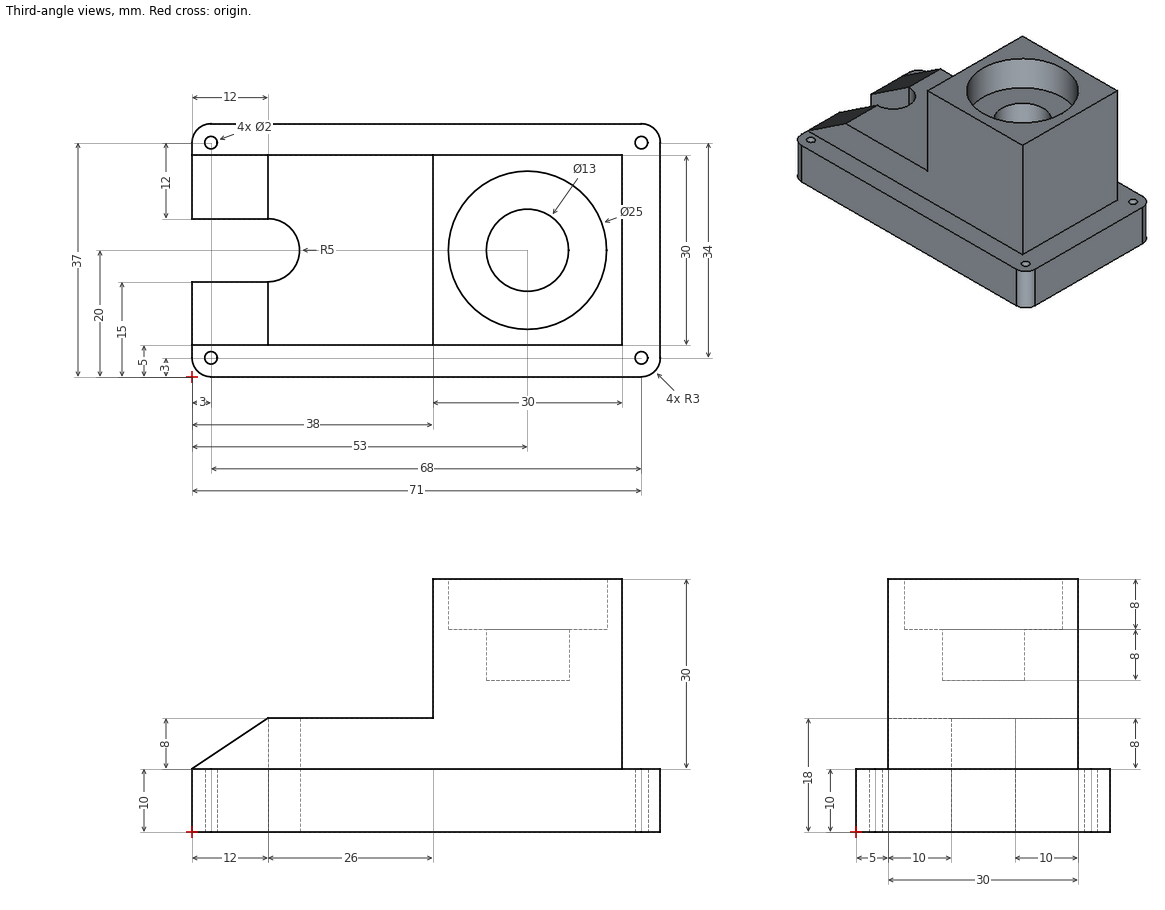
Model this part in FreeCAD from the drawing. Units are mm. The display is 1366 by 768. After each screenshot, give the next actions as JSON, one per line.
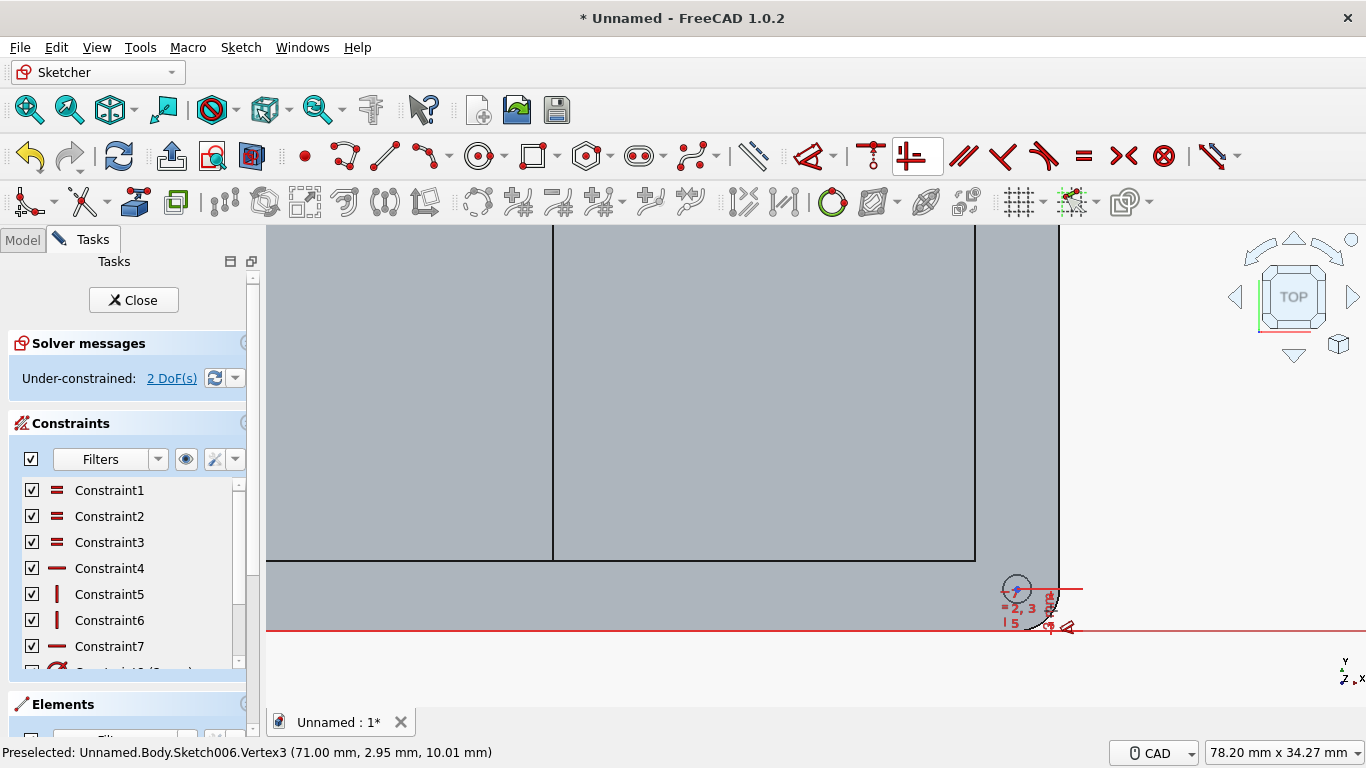
{"action": "scroll", "coordinate": [1018, 590], "scroll_direction": "down", "scroll_amount": 3}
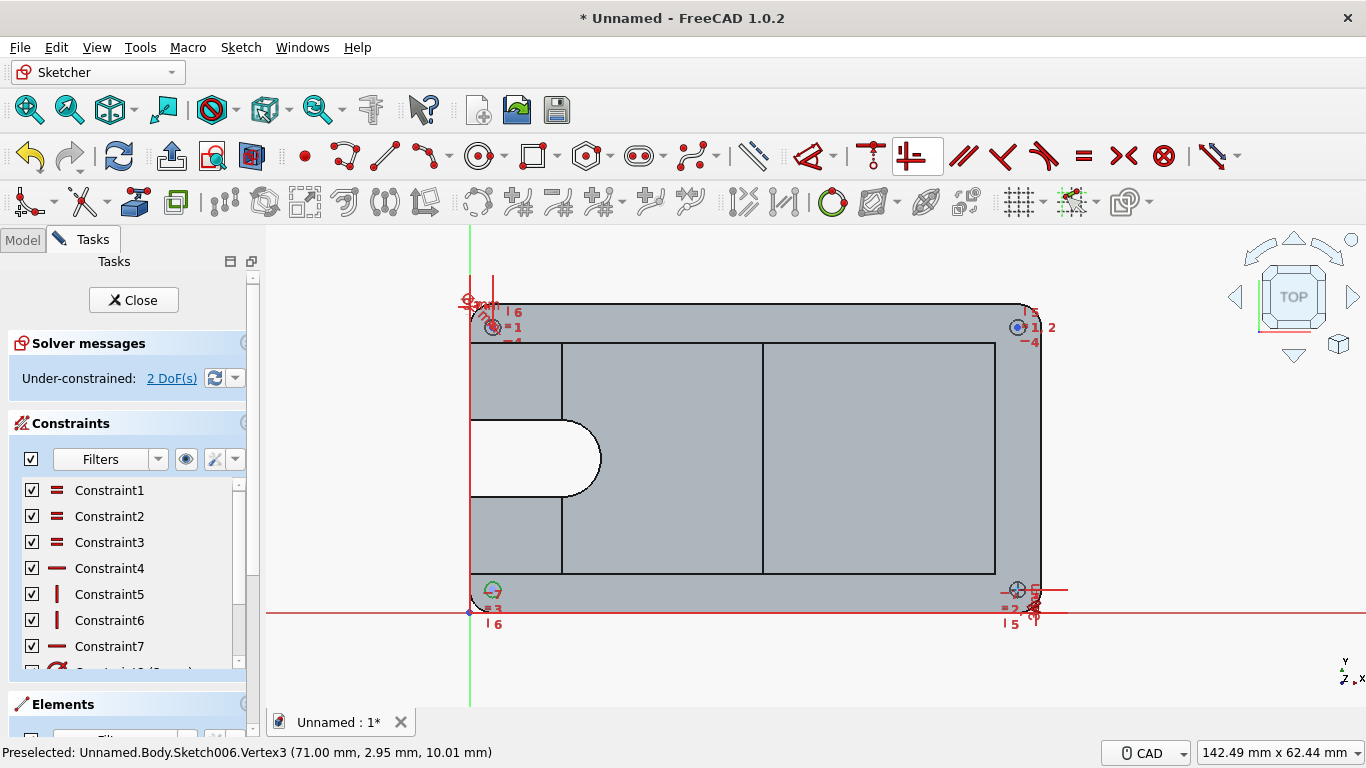
{"action": "left_click", "coordinate": [493, 328]}
{"action": "left_click", "coordinate": [436, 470]}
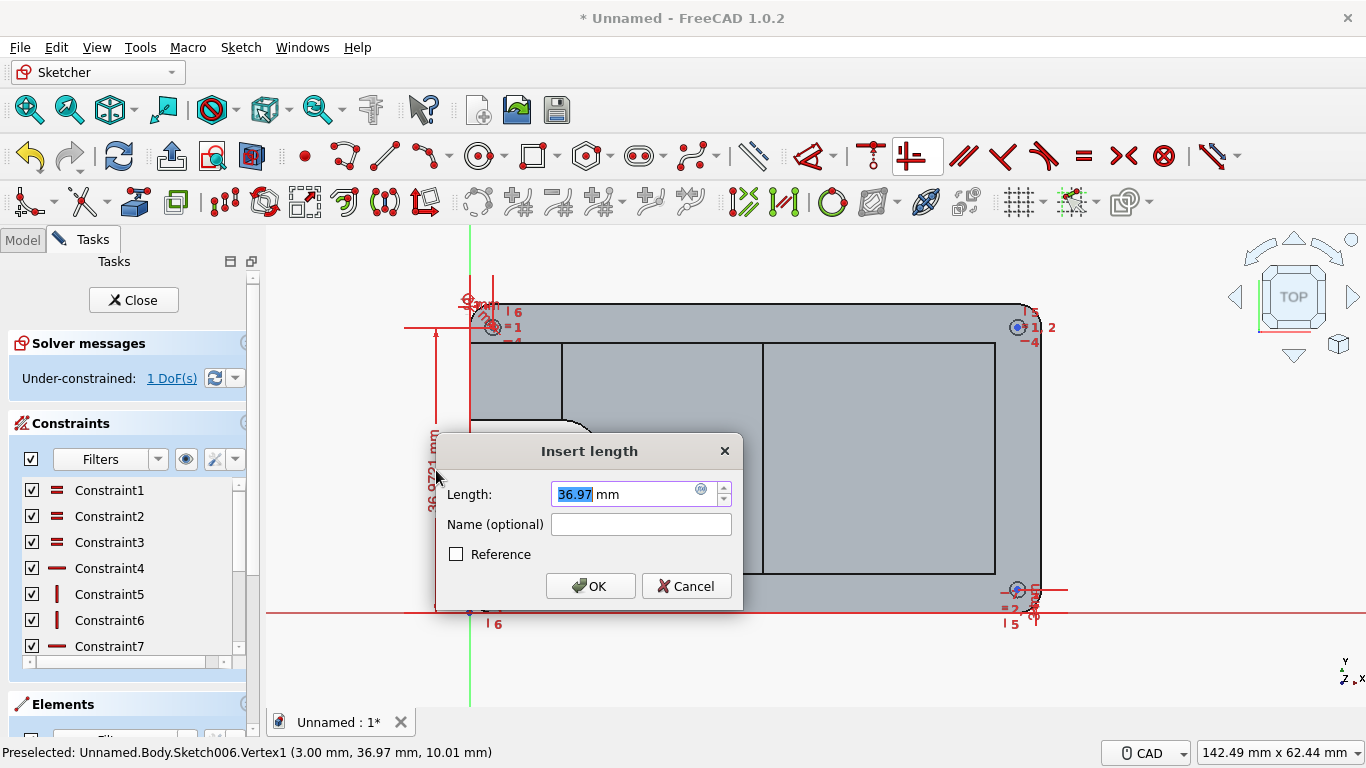
{"action": "type", "text": "37"}
{"action": "key", "text": "Return"}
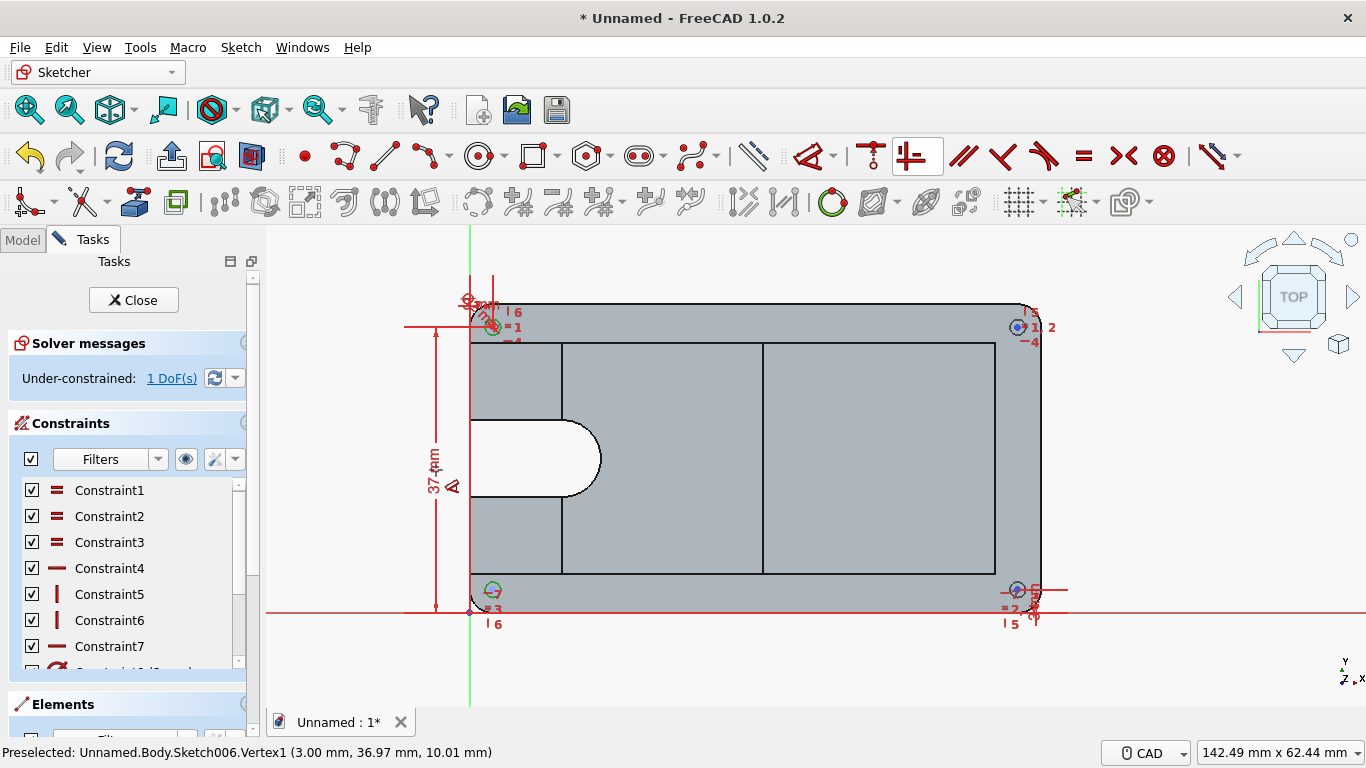
{"action": "left_click", "coordinate": [1018, 327]}
{"action": "left_click", "coordinate": [744, 647]}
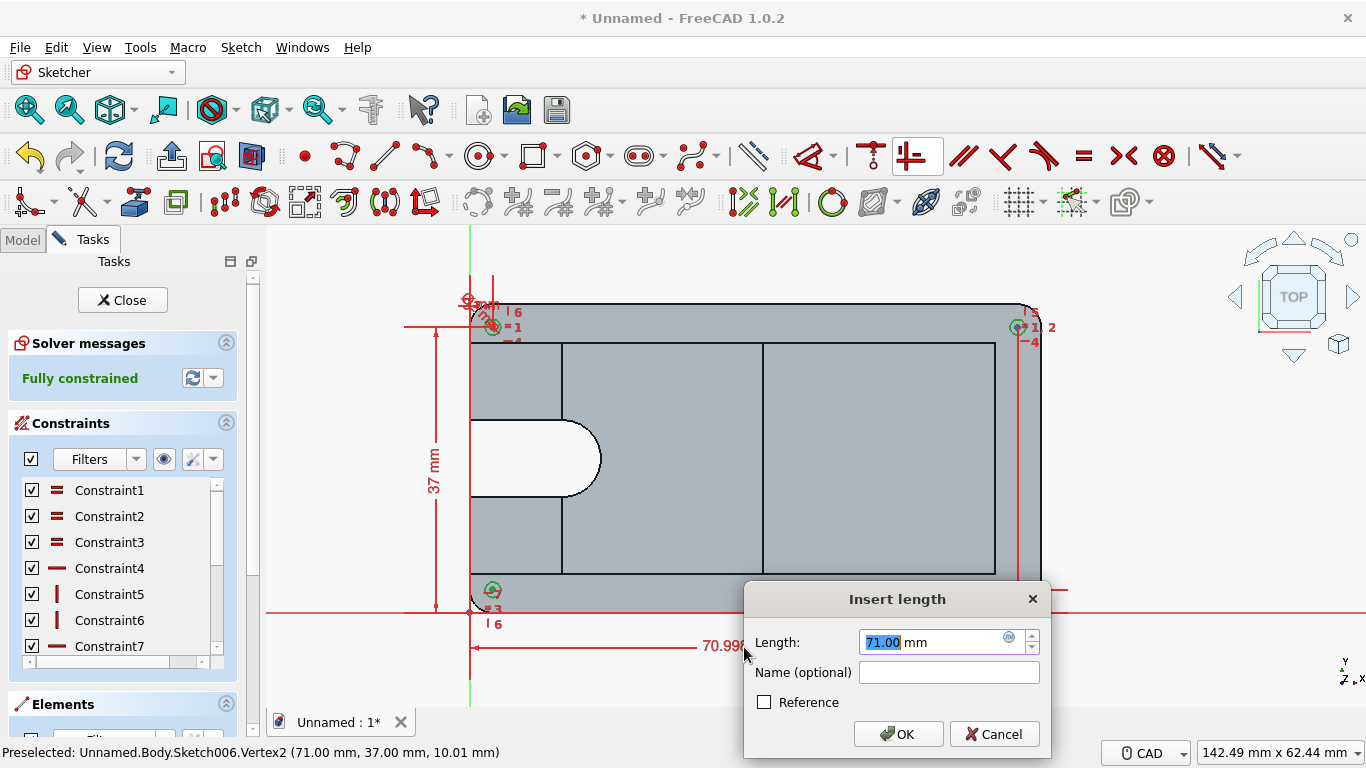
{"action": "type", "text": "71"}
{"action": "key", "text": "Return"}
{"action": "key", "text": "Escape"}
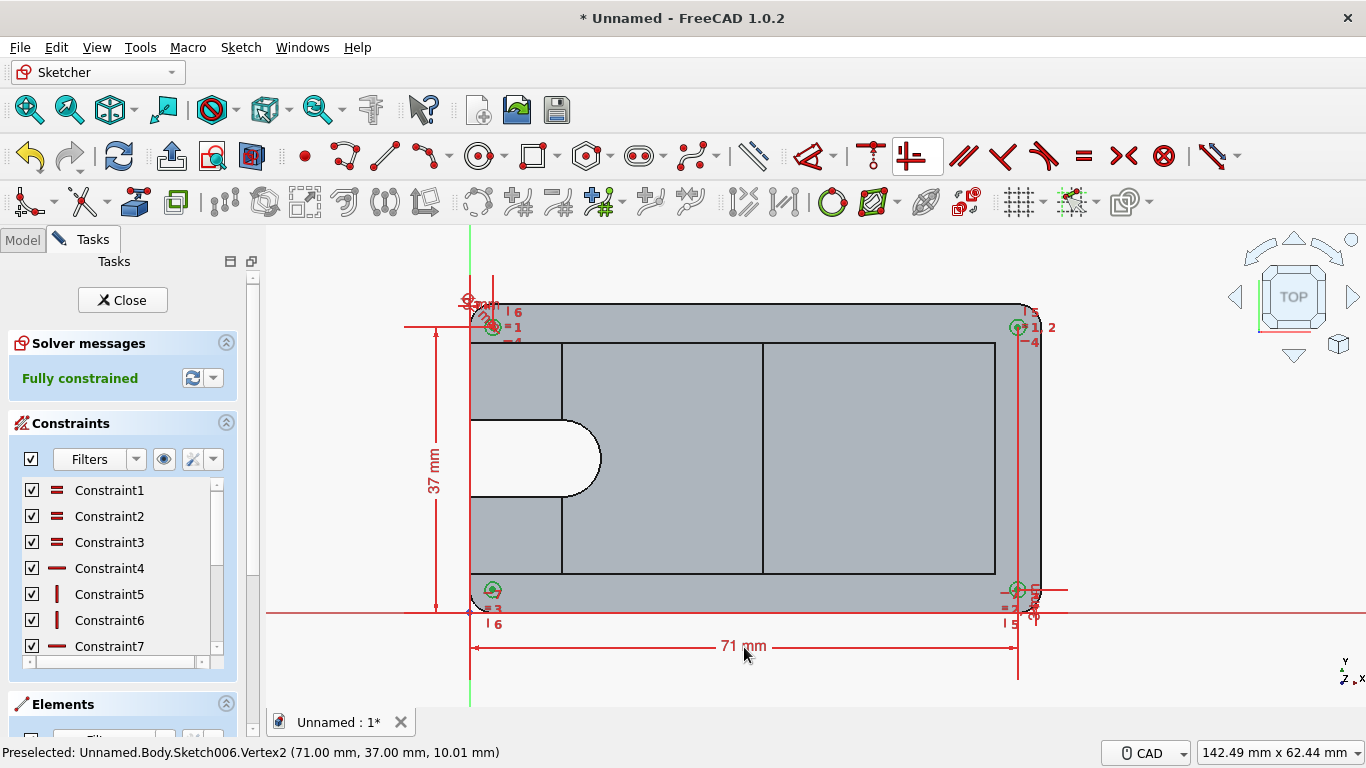
{"action": "left_click", "coordinate": [123, 300]}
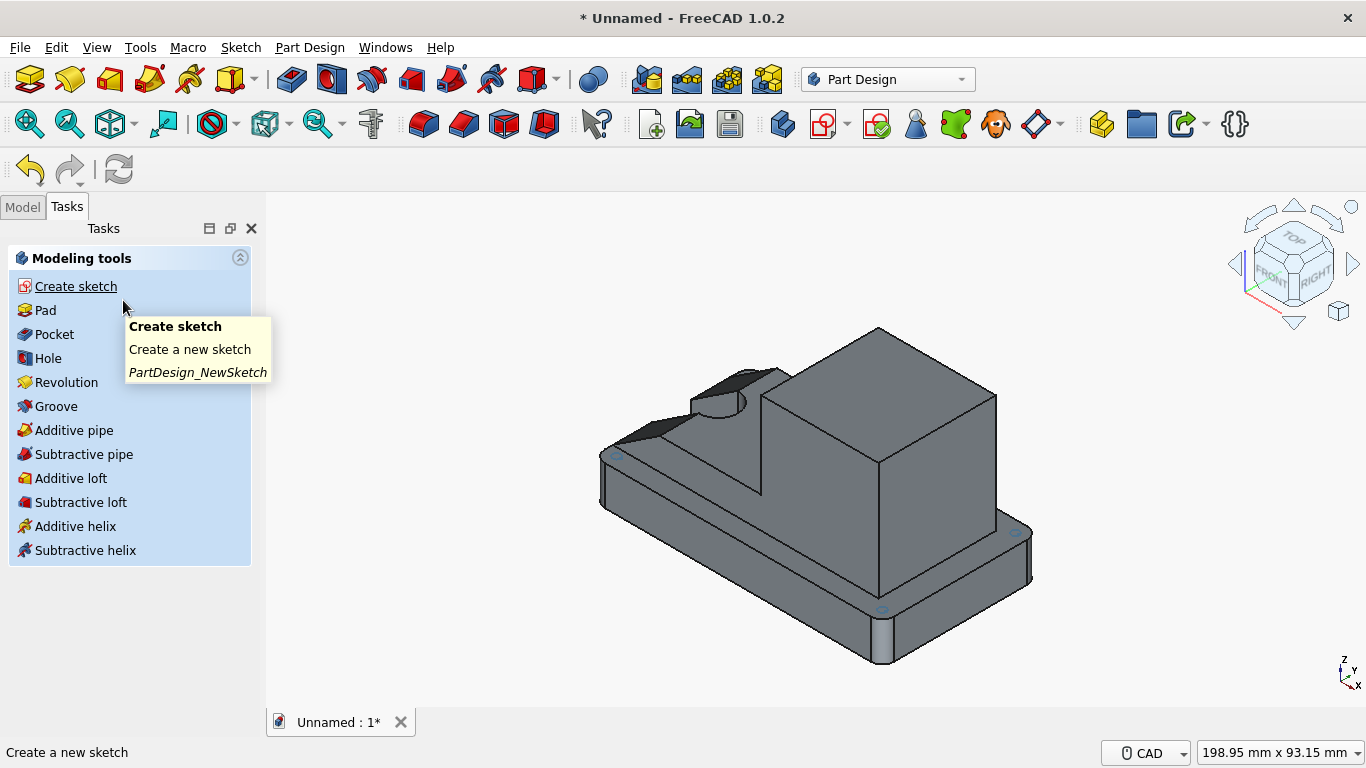
{"action": "left_click", "coordinate": [292, 80]}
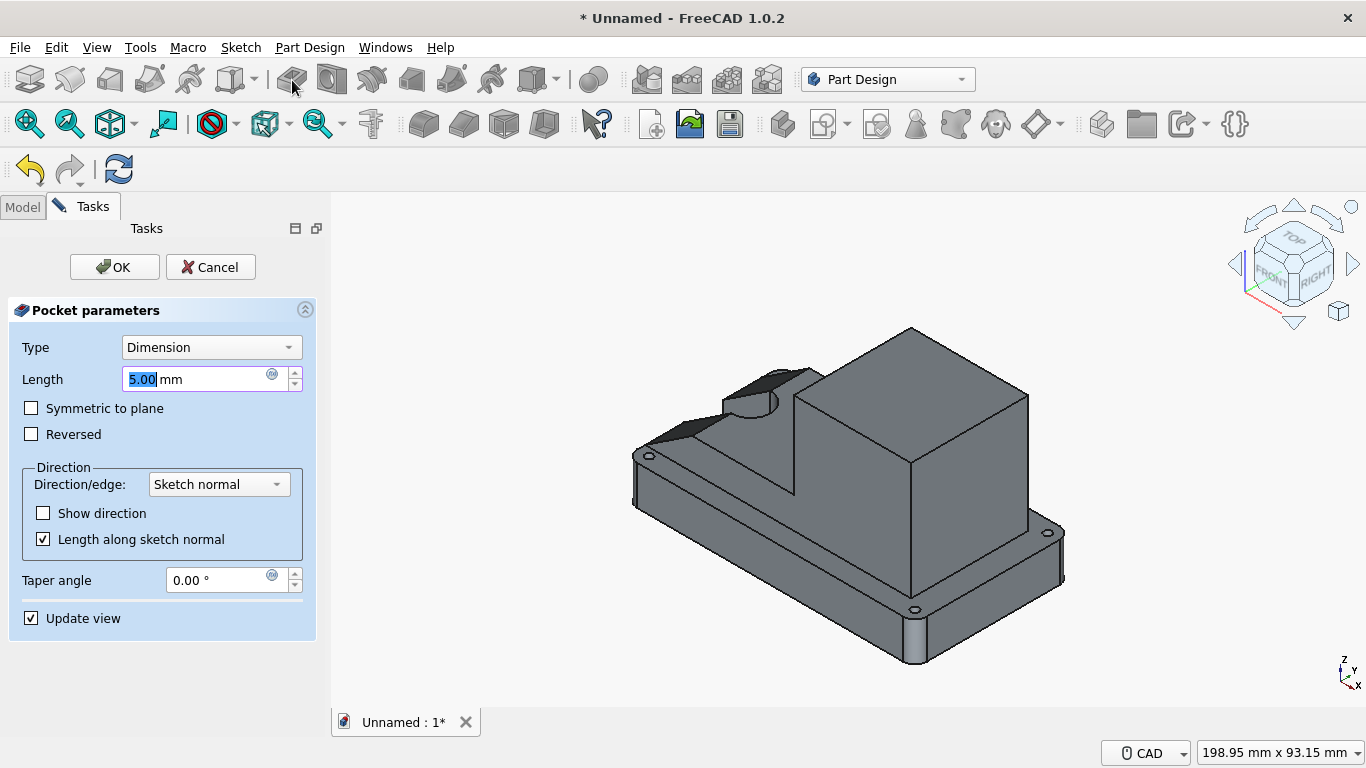
{"action": "type", "text": "10"}
{"action": "key", "text": "Tab"}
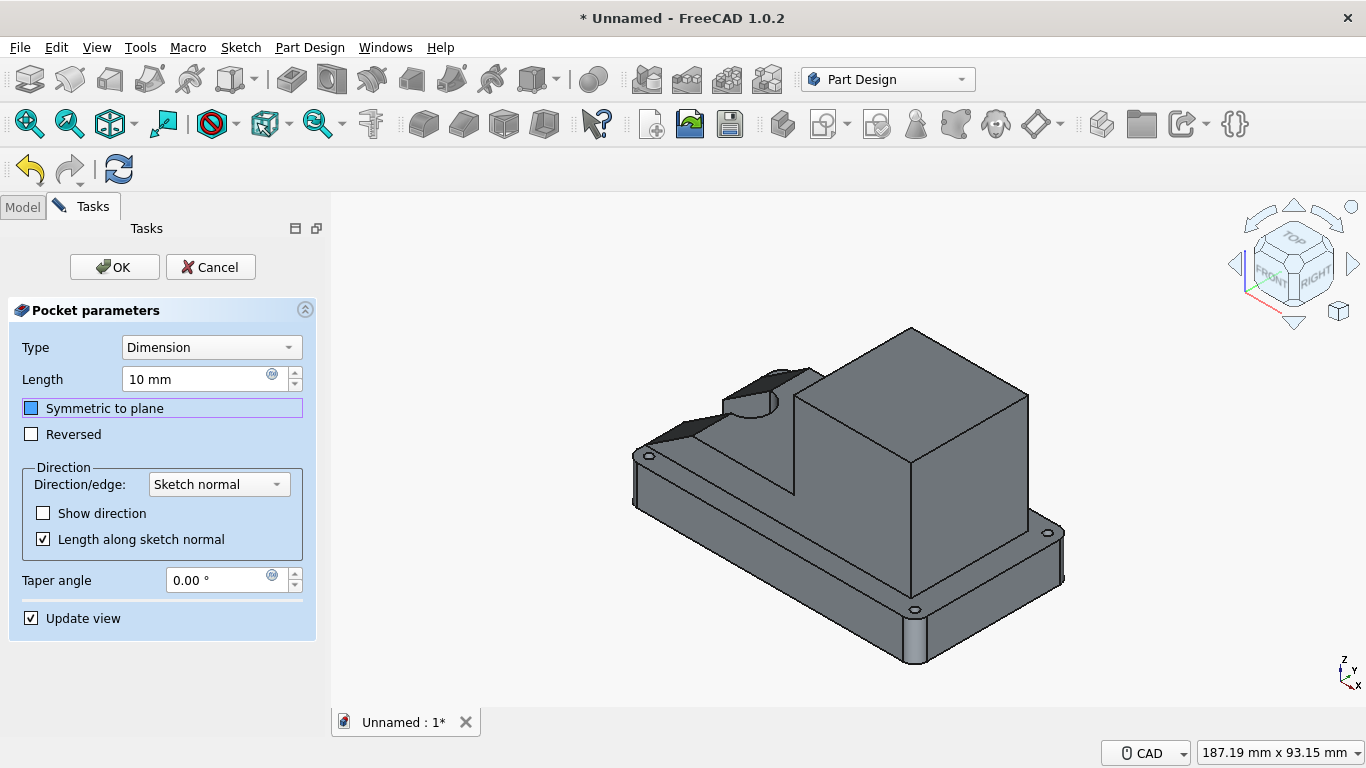
{"action": "left_click", "coordinate": [115, 267]}